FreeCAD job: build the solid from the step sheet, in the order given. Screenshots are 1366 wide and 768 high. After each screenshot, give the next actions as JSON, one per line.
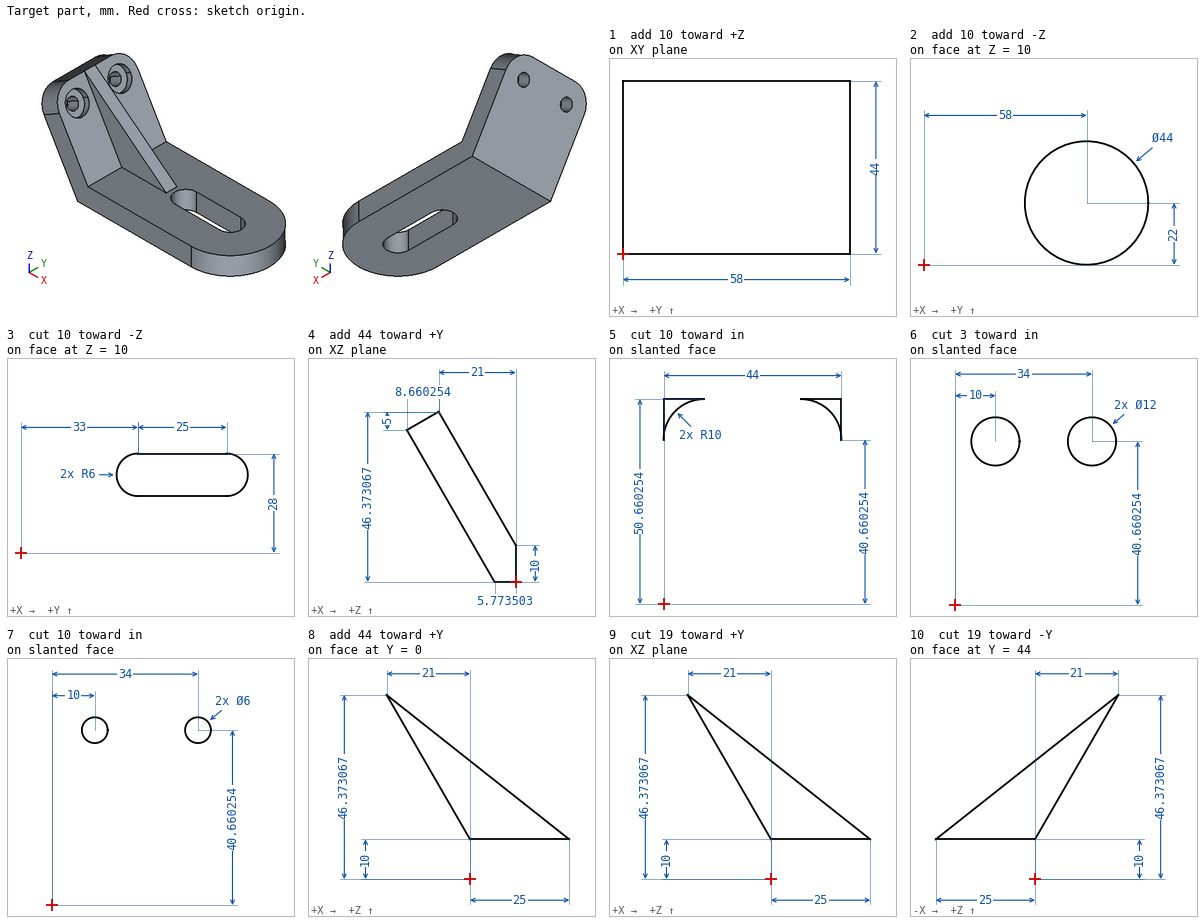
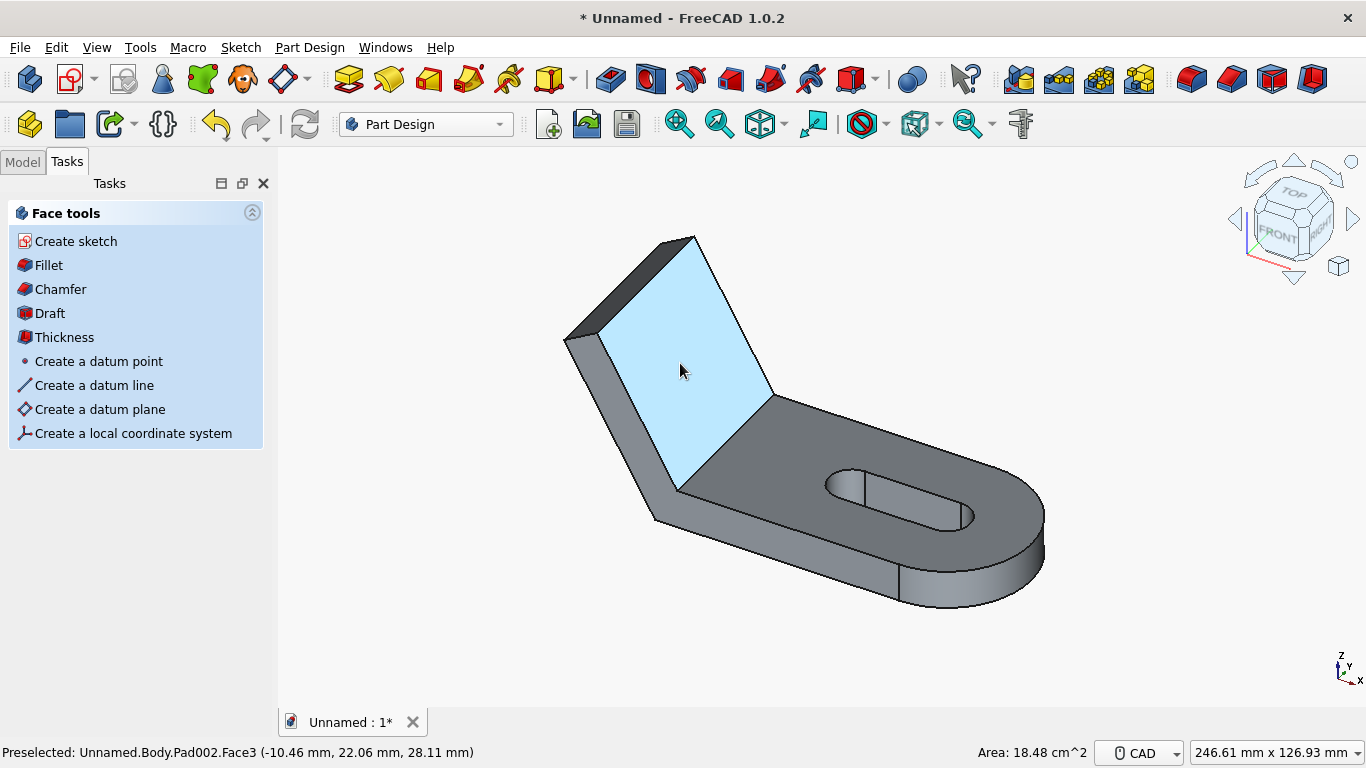
{"action": "left_click", "coordinate": [70, 80]}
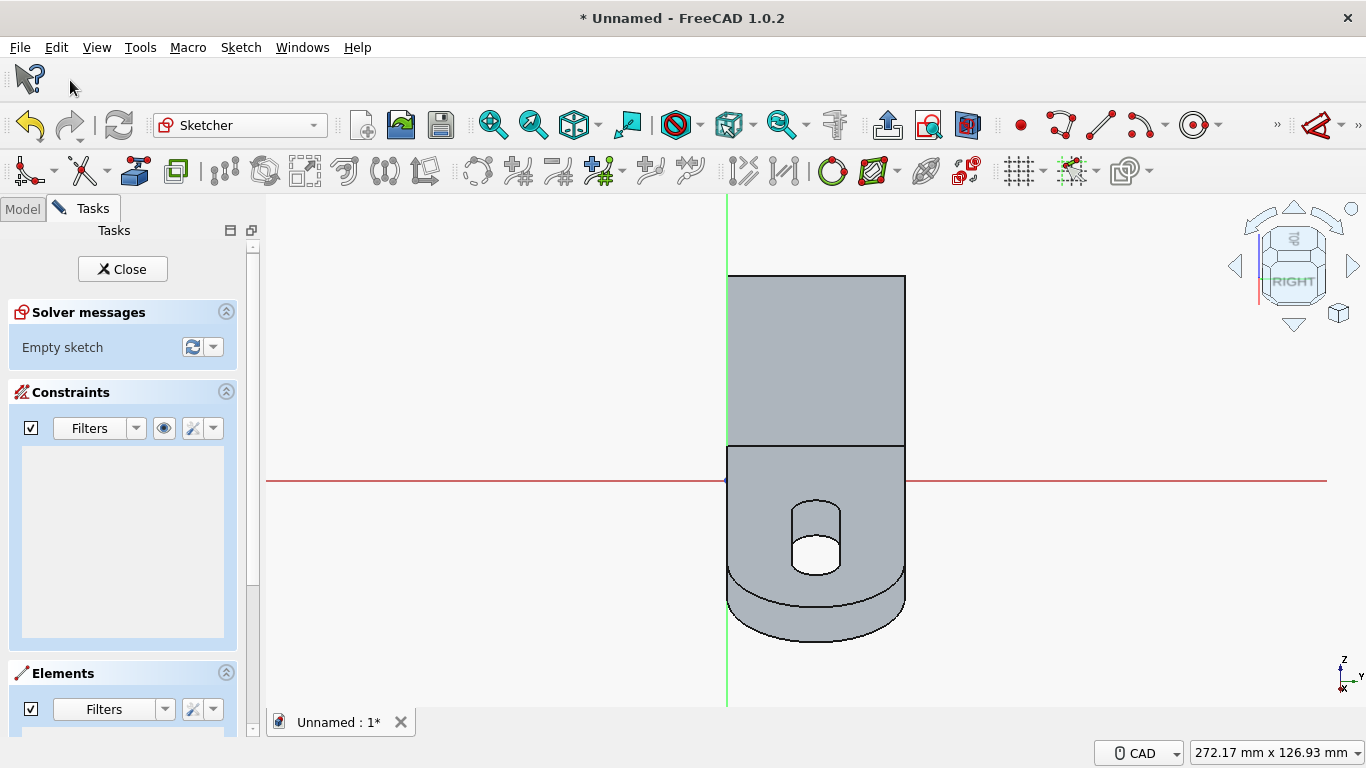
{"action": "left_click", "coordinate": [968, 126]}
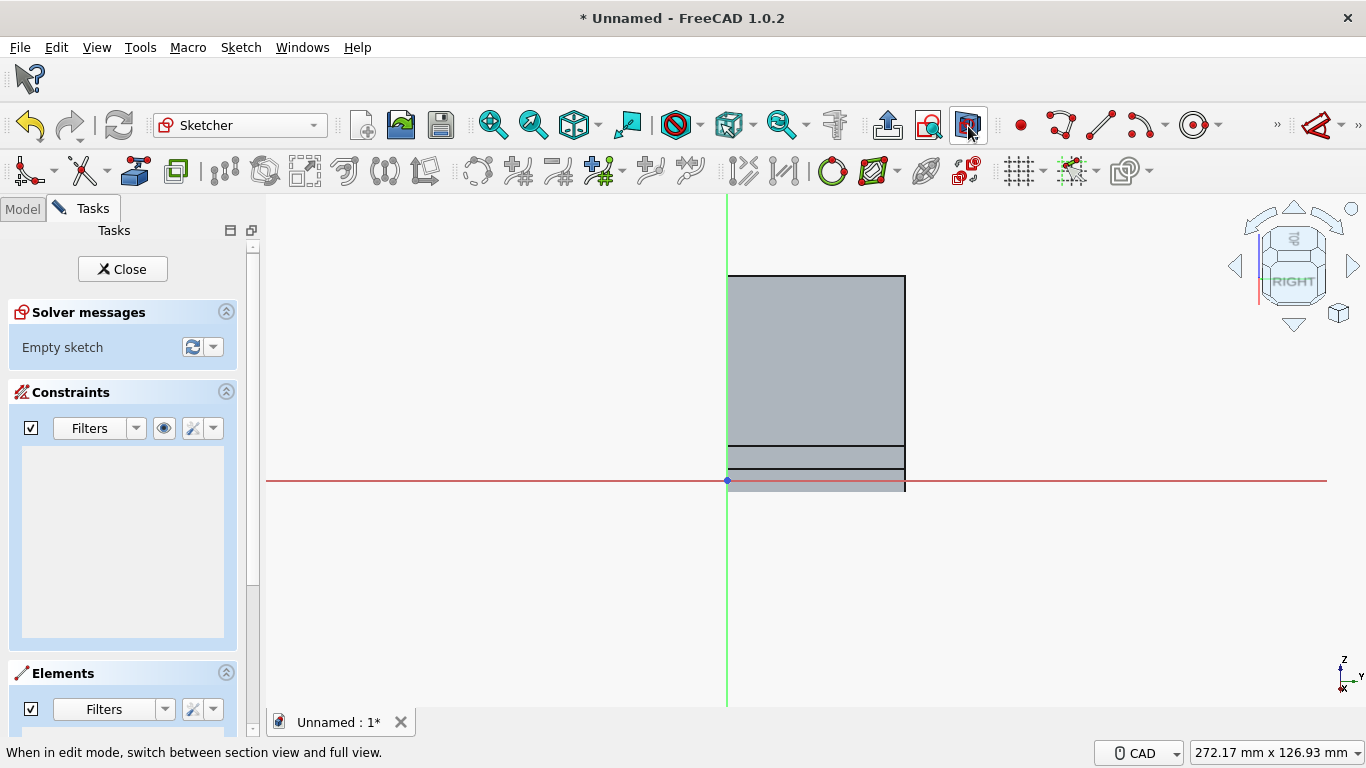
{"action": "scroll", "coordinate": [955, 232], "scroll_direction": "up", "scroll_amount": 2}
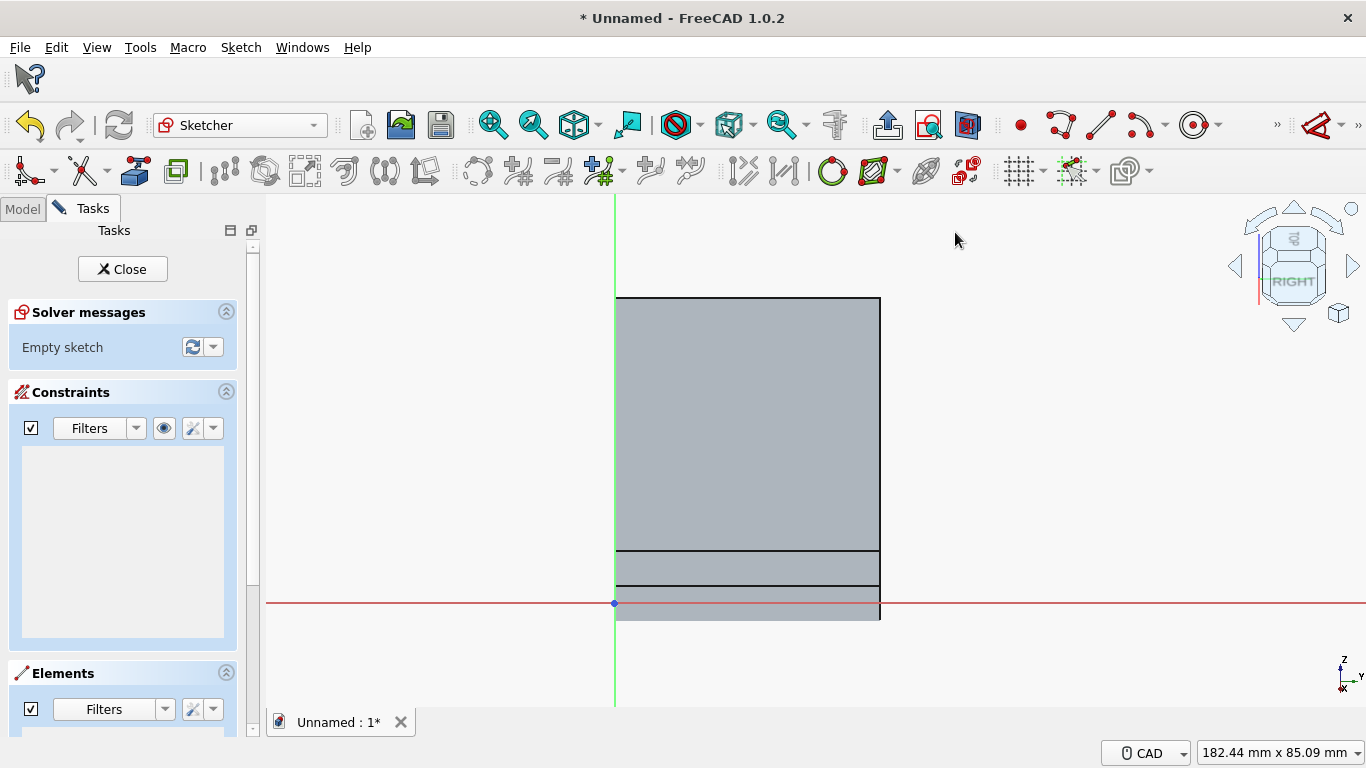
{"action": "left_click", "coordinate": [1062, 126]}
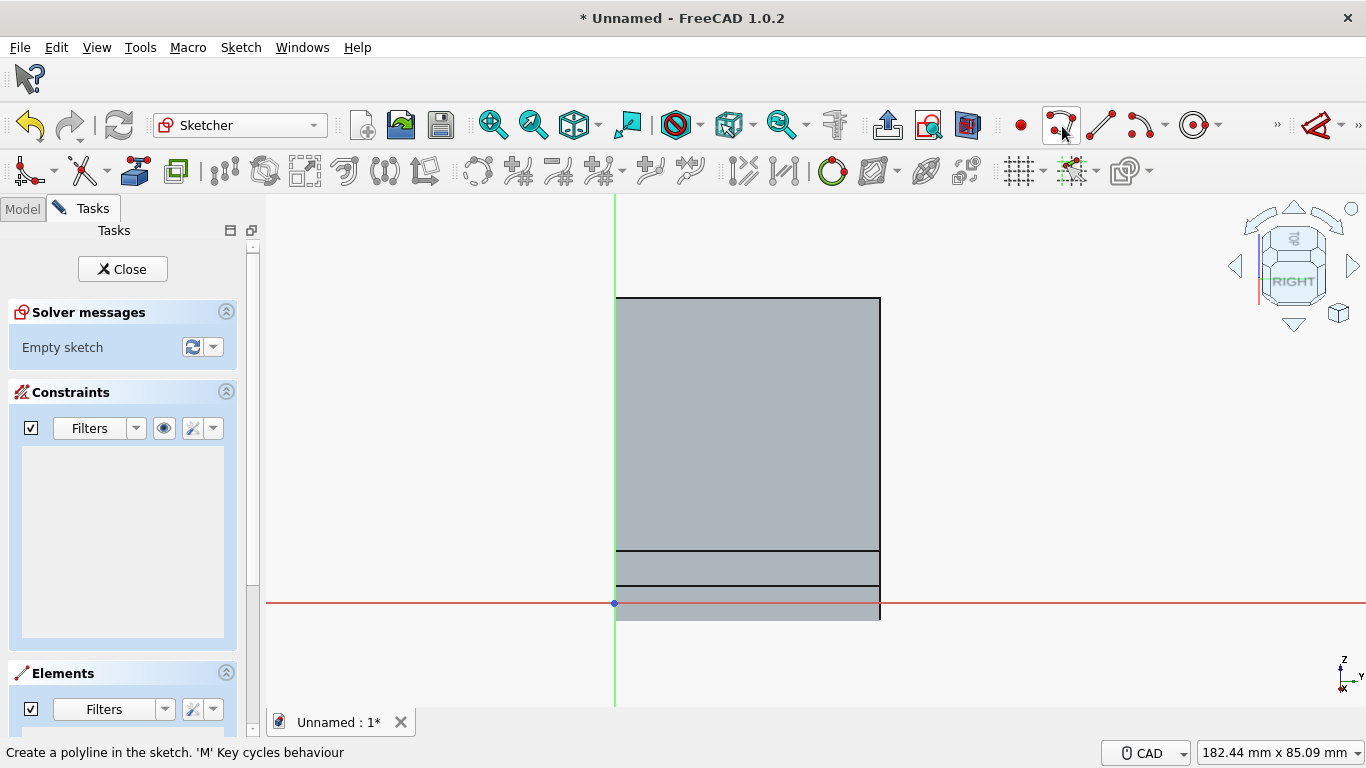
{"action": "left_click", "coordinate": [675, 298]}
{"action": "left_click", "coordinate": [615, 298]}
{"action": "left_click", "coordinate": [624, 358]}
{"action": "right_click", "coordinate": [624, 358]}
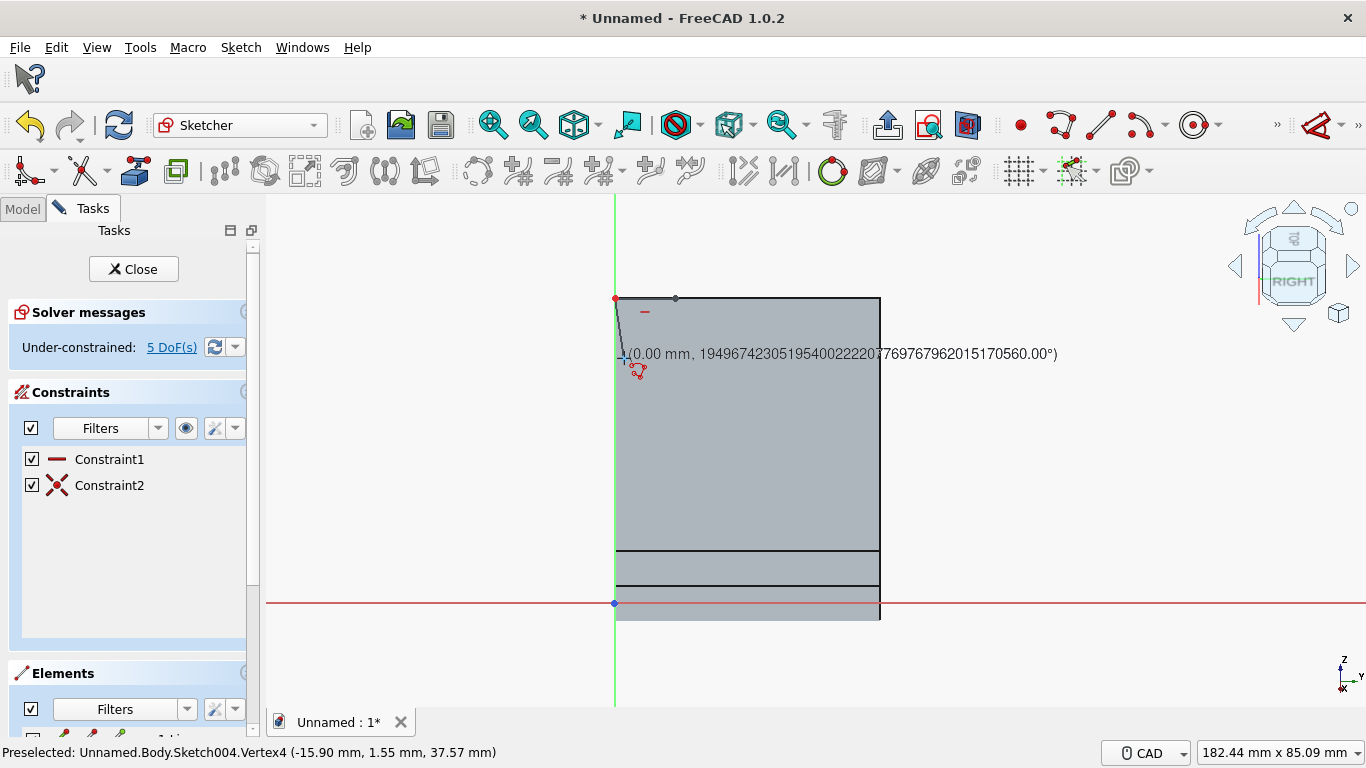
{"action": "left_click", "coordinate": [1168, 126]}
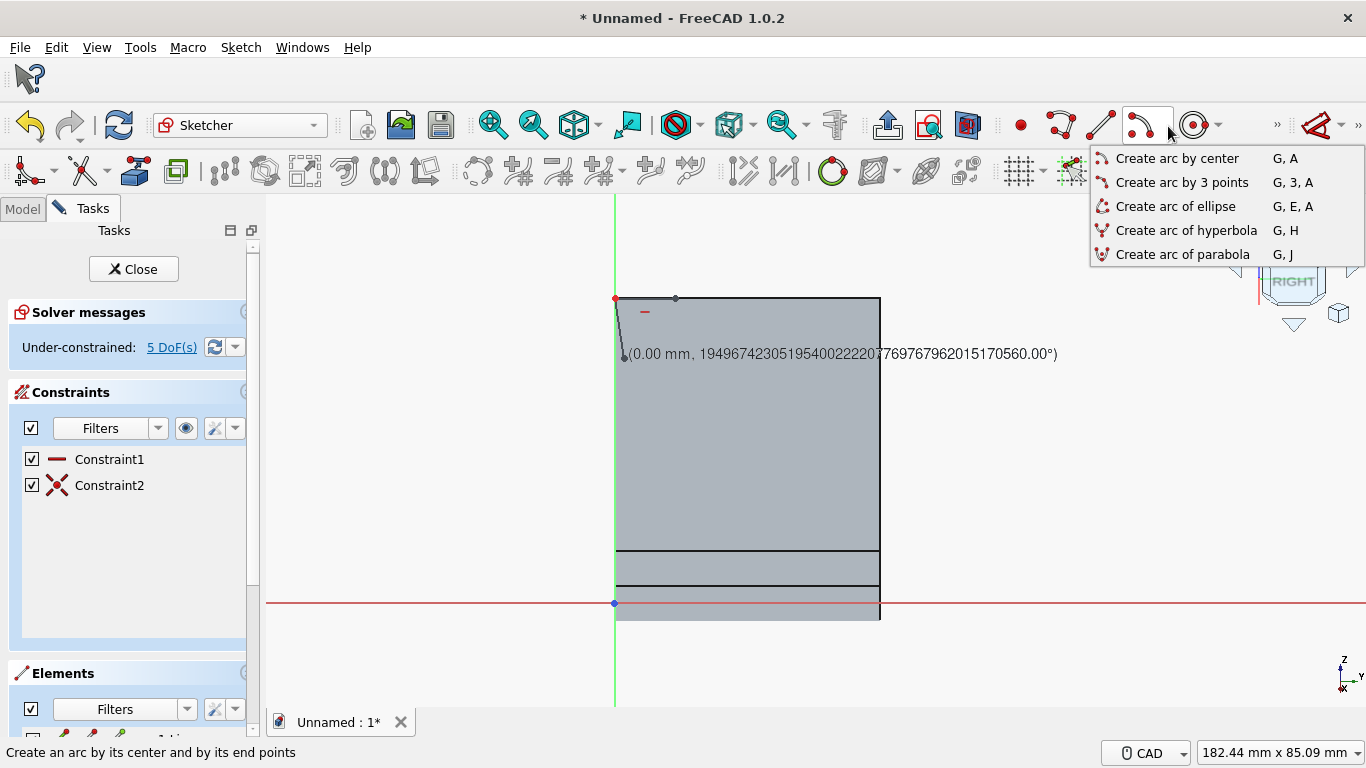
{"action": "left_click", "coordinate": [1228, 182]}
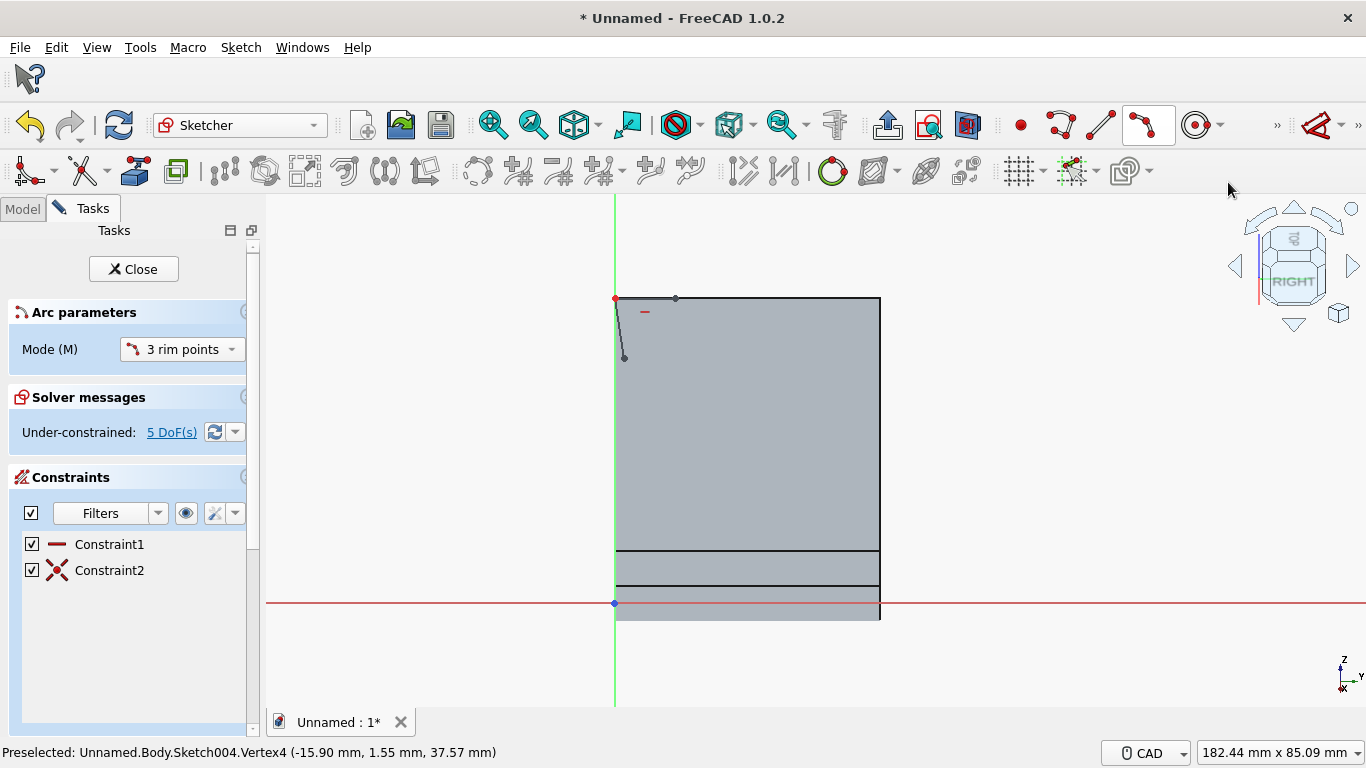
{"action": "left_click", "coordinate": [624, 359]}
{"action": "left_click", "coordinate": [675, 299]}
{"action": "left_click", "coordinate": [632, 315]}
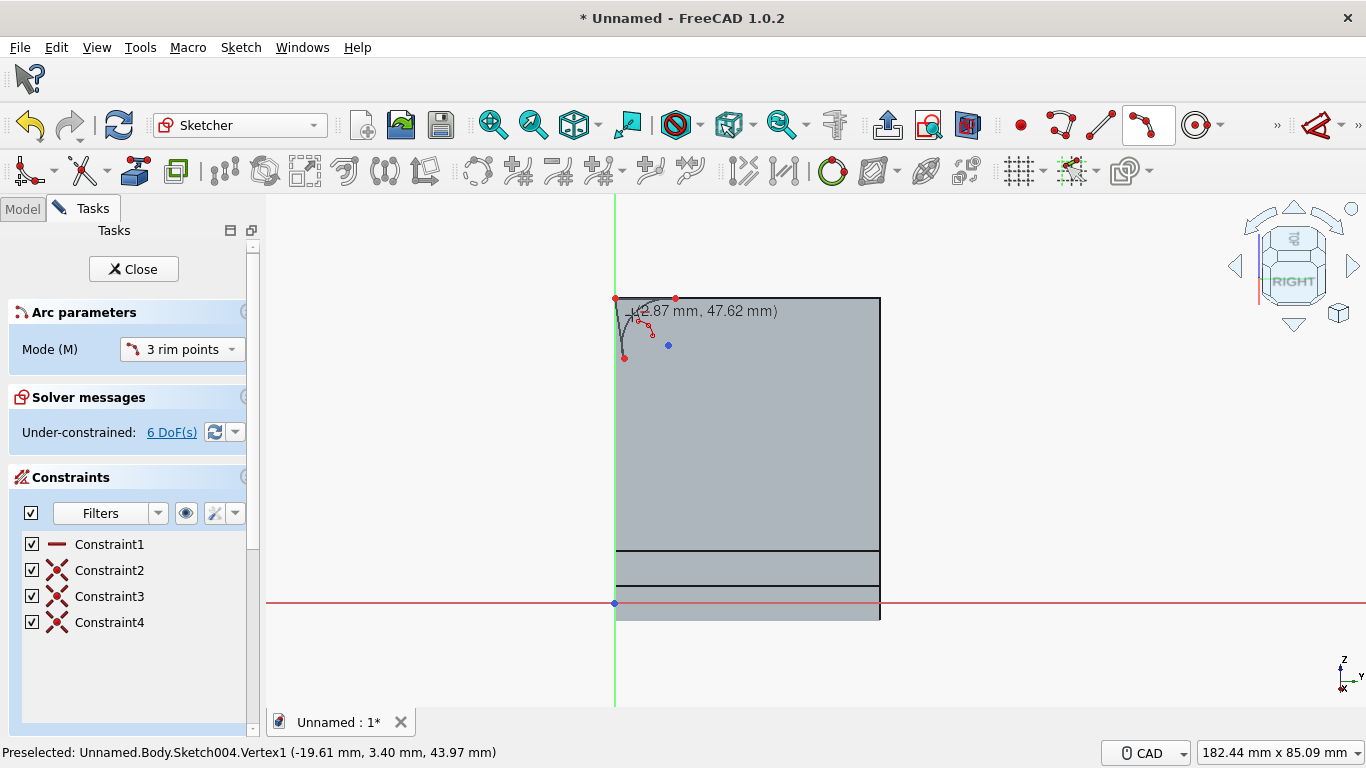
{"action": "left_click", "coordinate": [1062, 126]}